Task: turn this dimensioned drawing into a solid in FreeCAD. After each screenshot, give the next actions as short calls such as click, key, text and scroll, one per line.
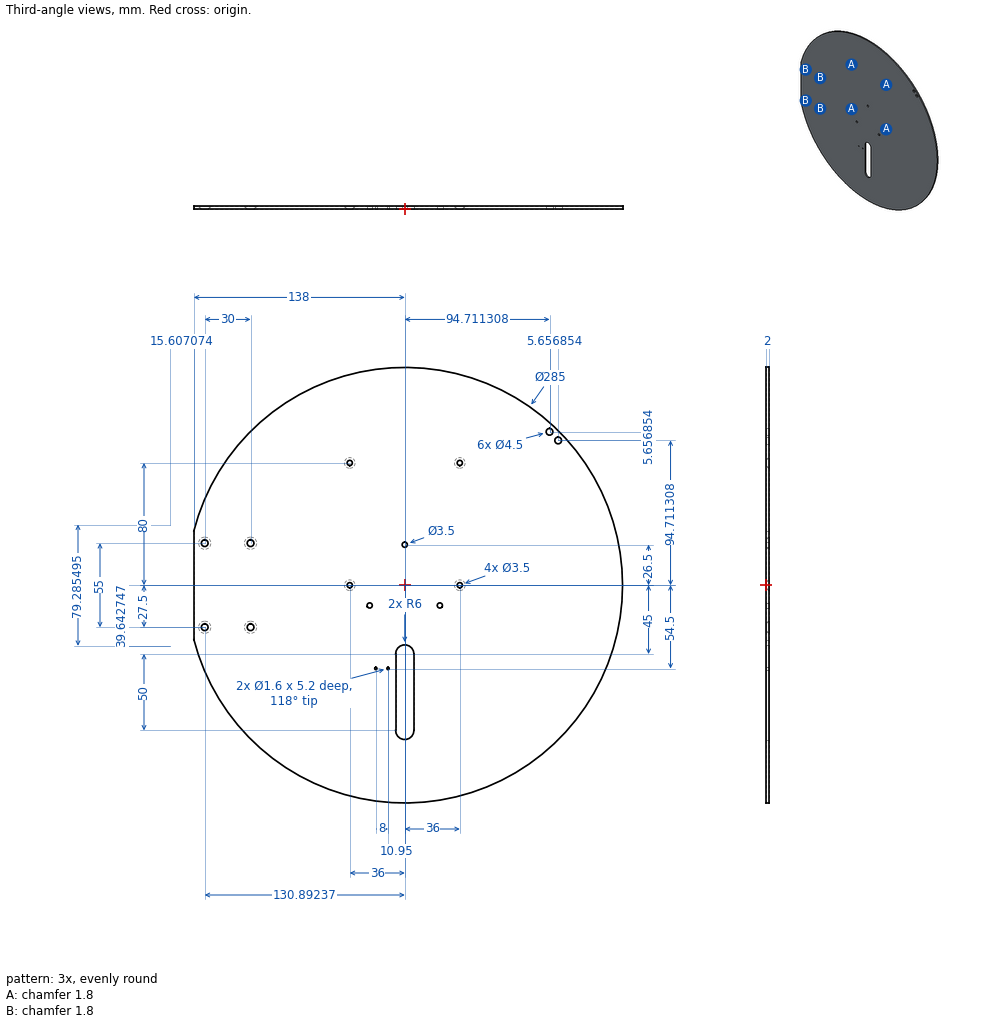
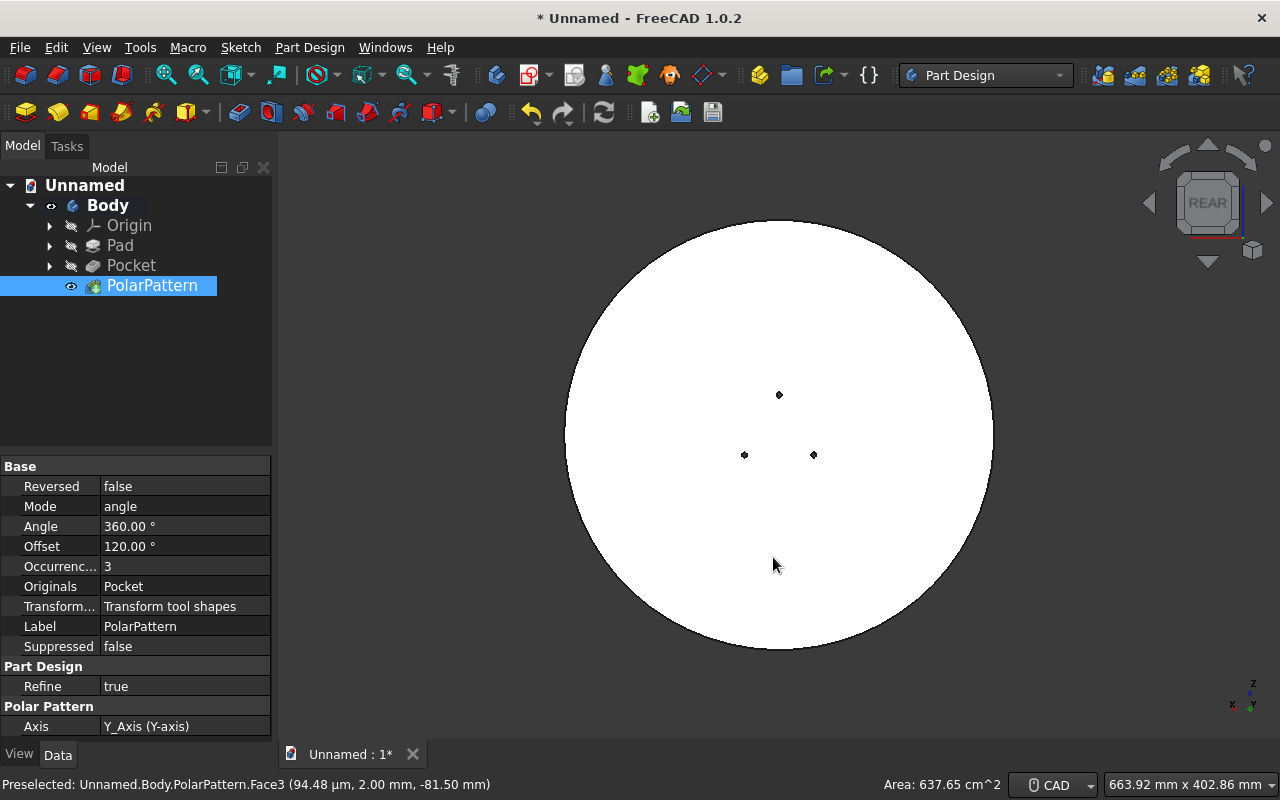
click(530, 76)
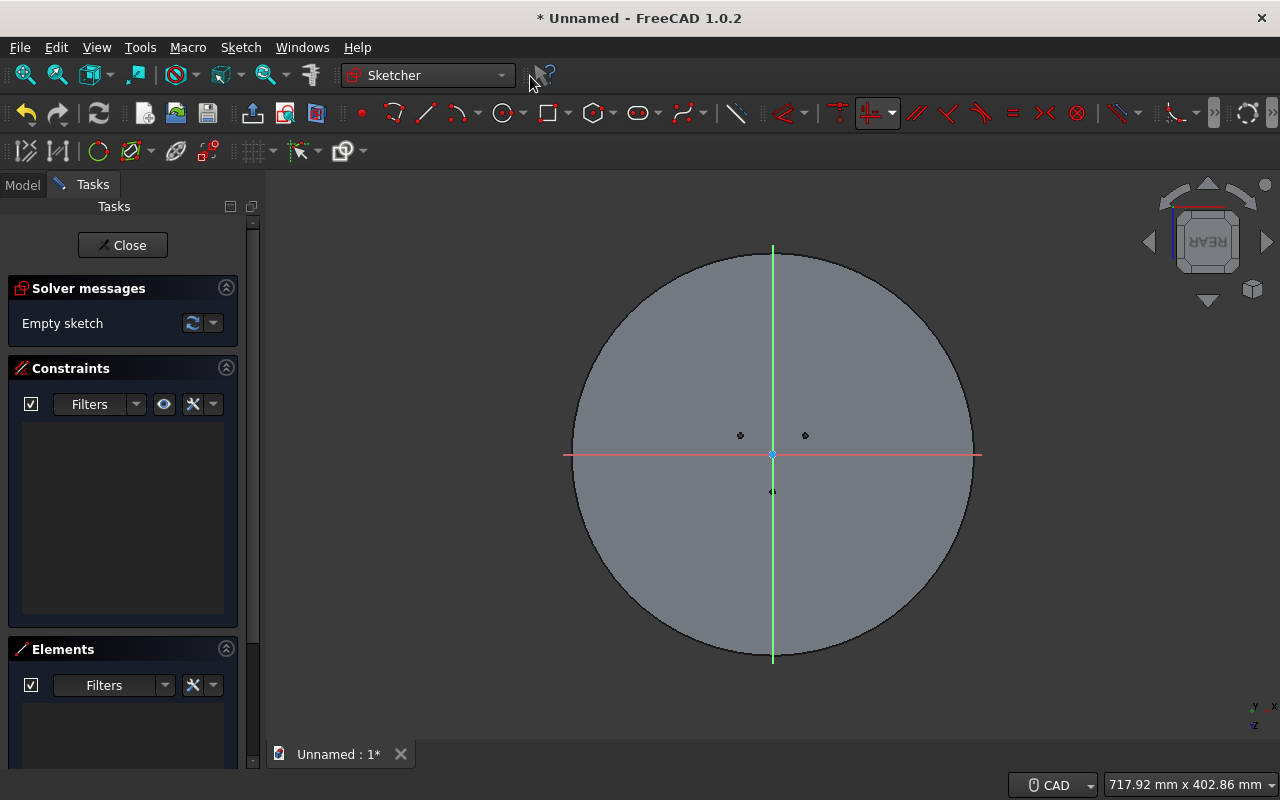
scroll(808, 569, up, 3)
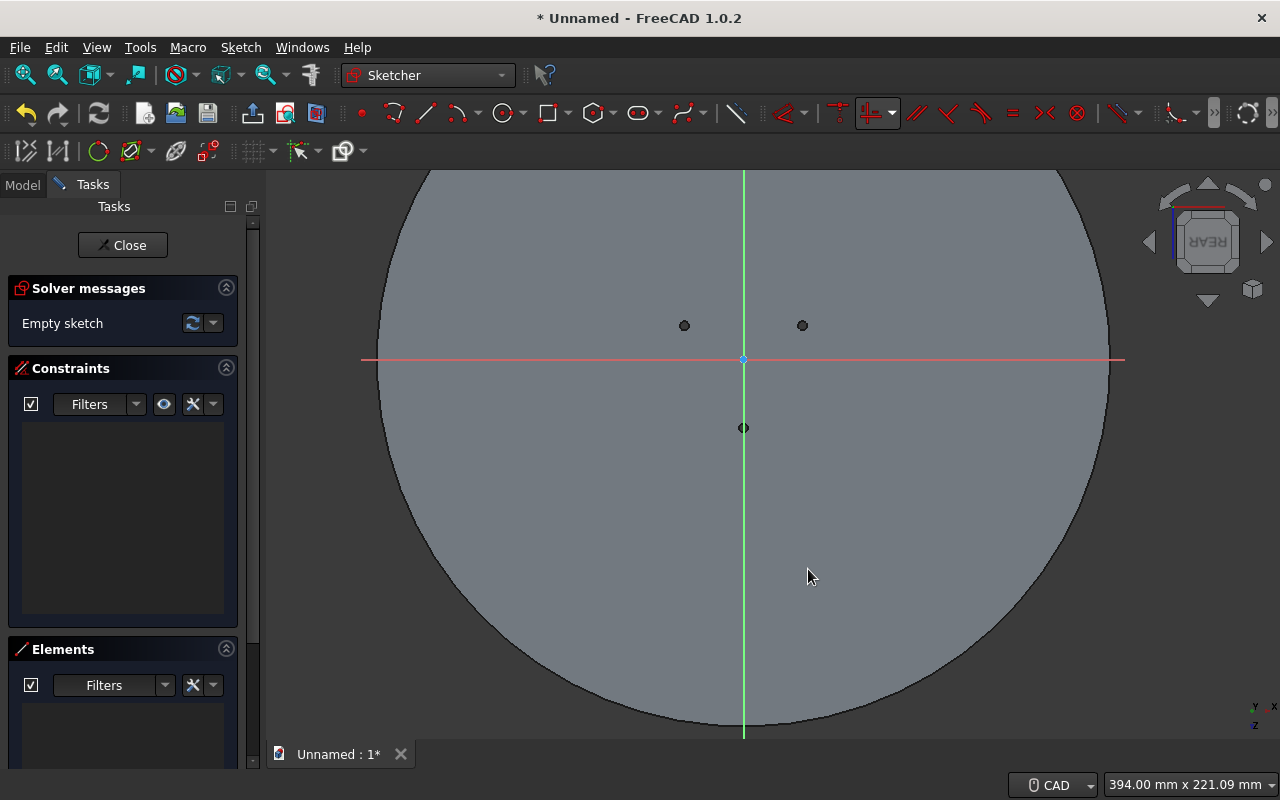
click(504, 114)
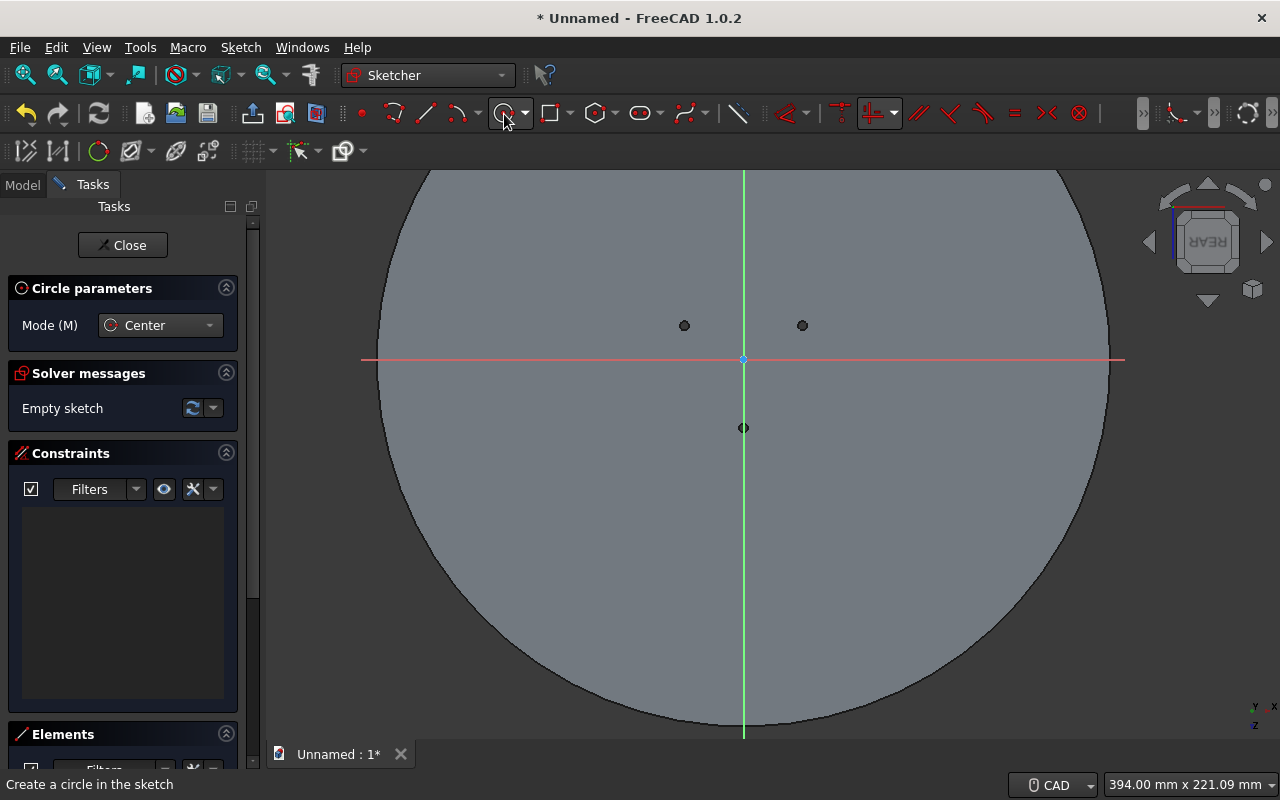
scroll(987, 618, up, 7)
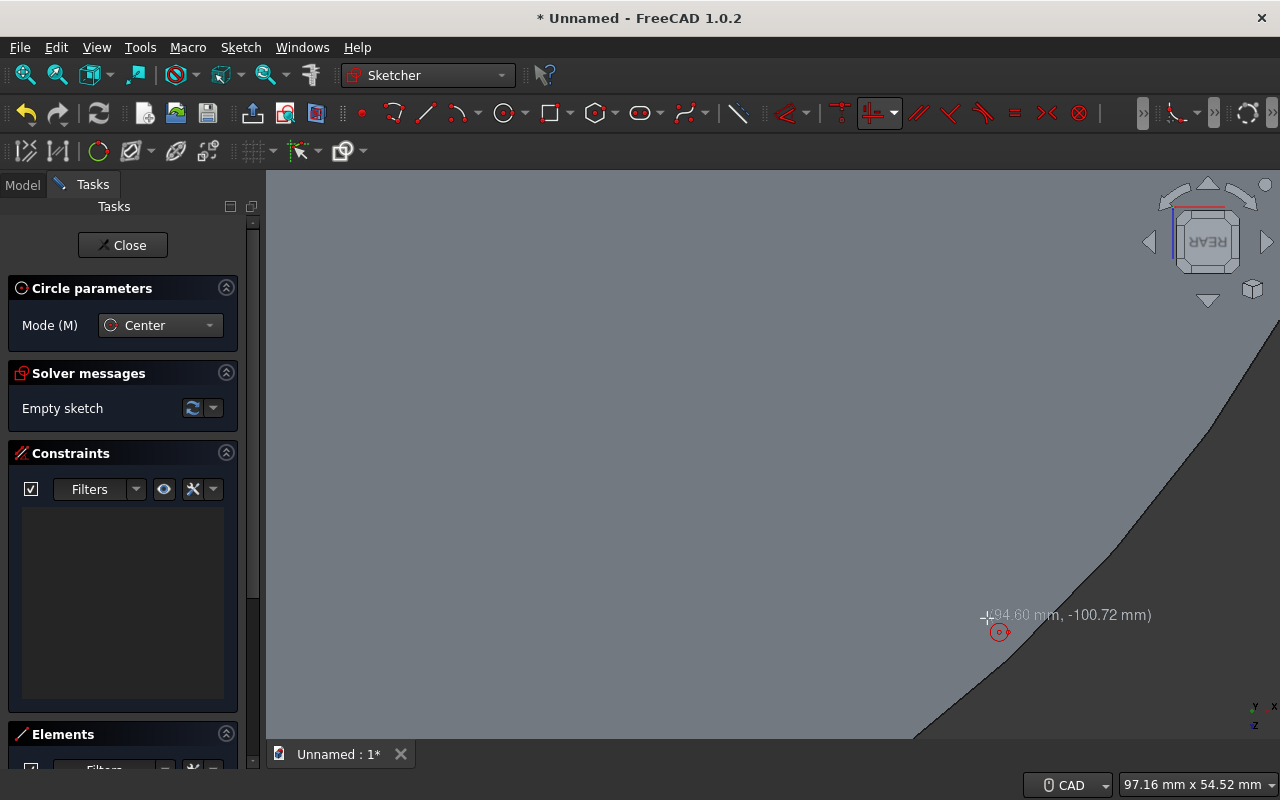
scroll(988, 620, down, 7)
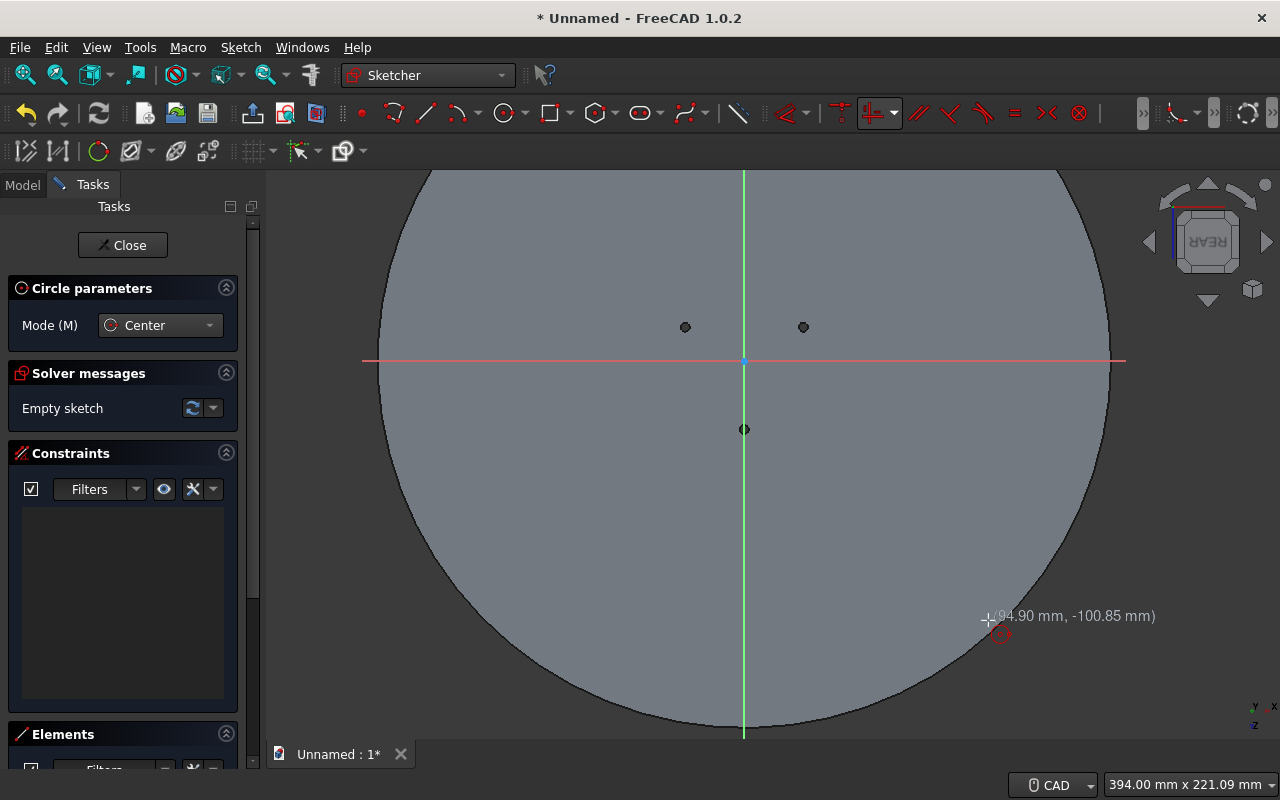
click(988, 620)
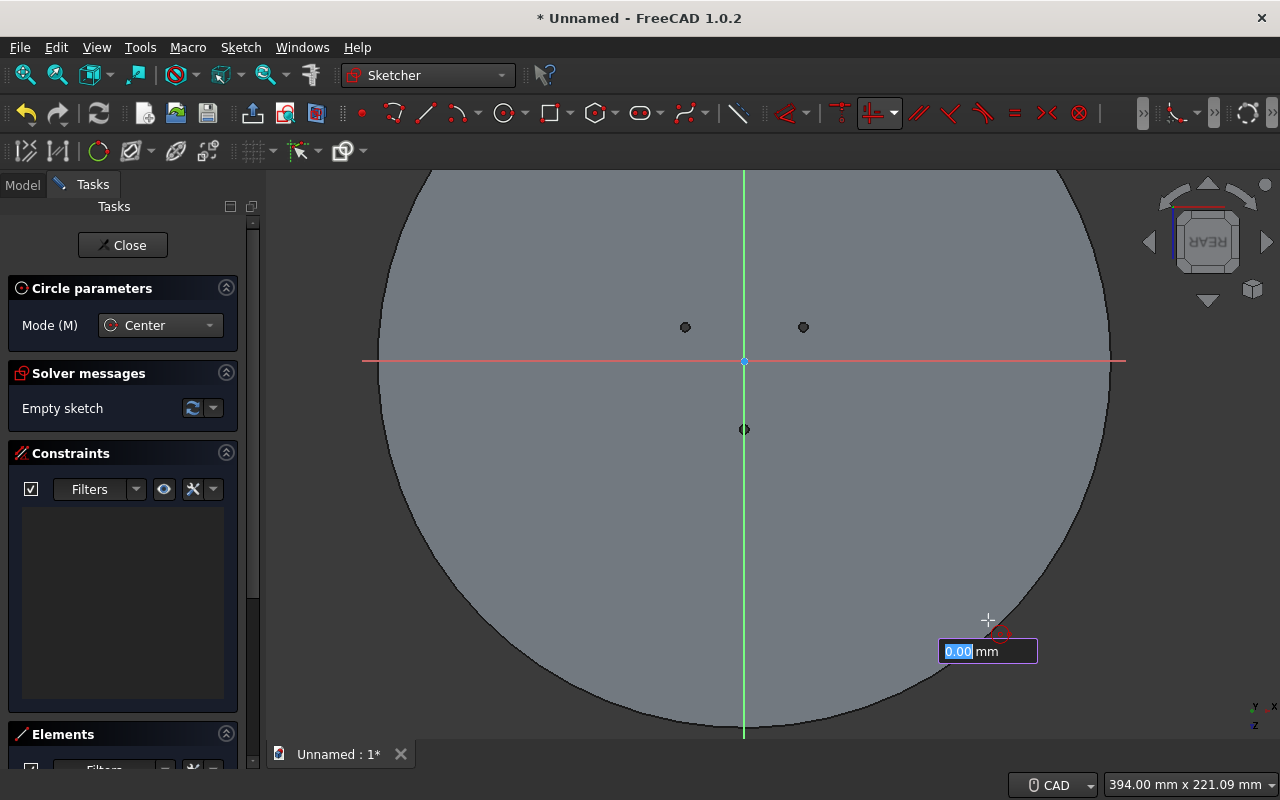
scroll(992, 616, up, 6)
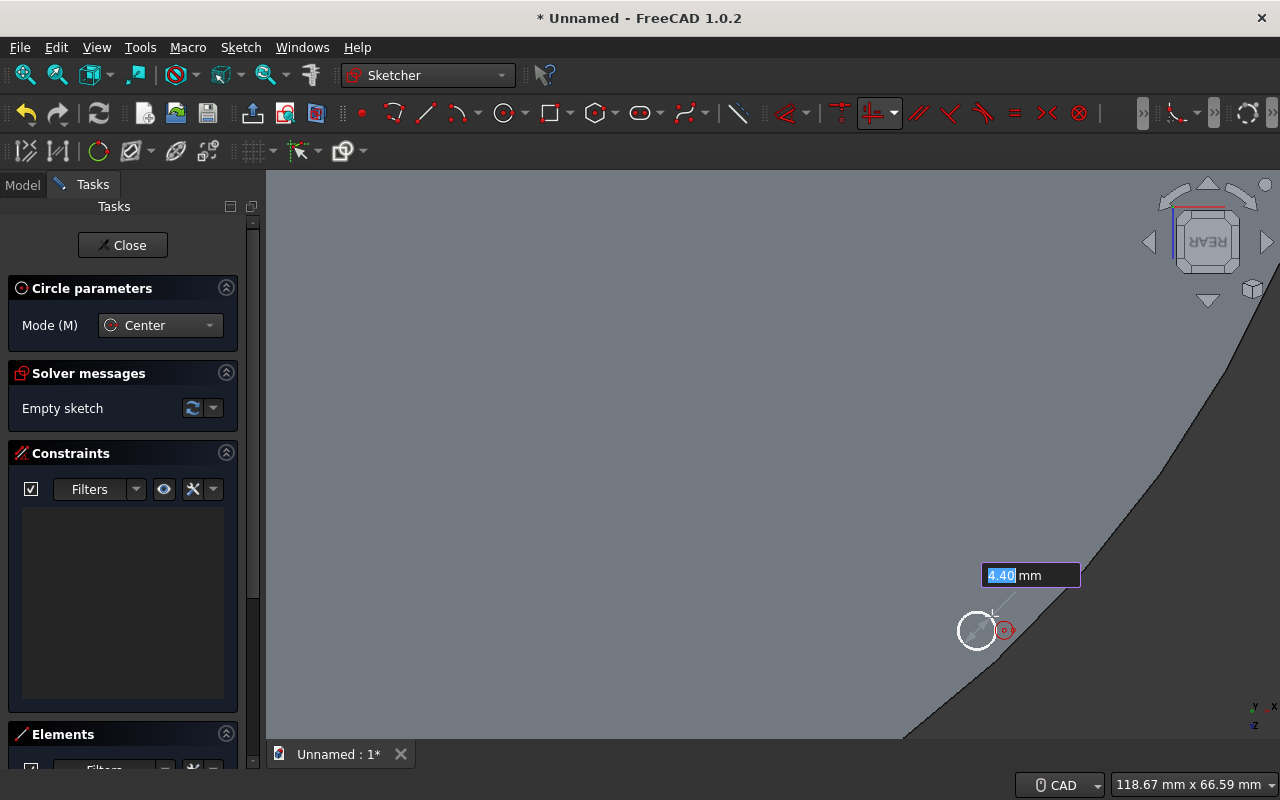
click(991, 613)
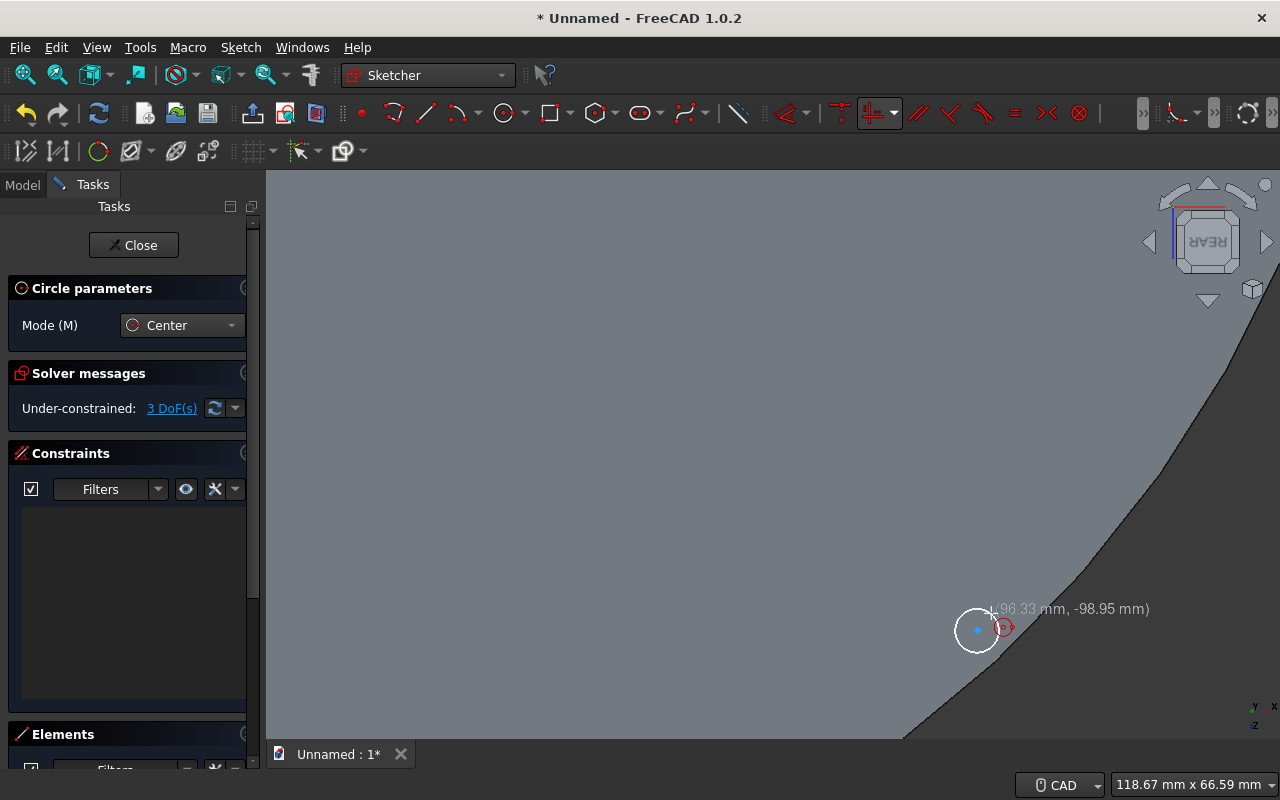
click(1026, 578)
click(1039, 564)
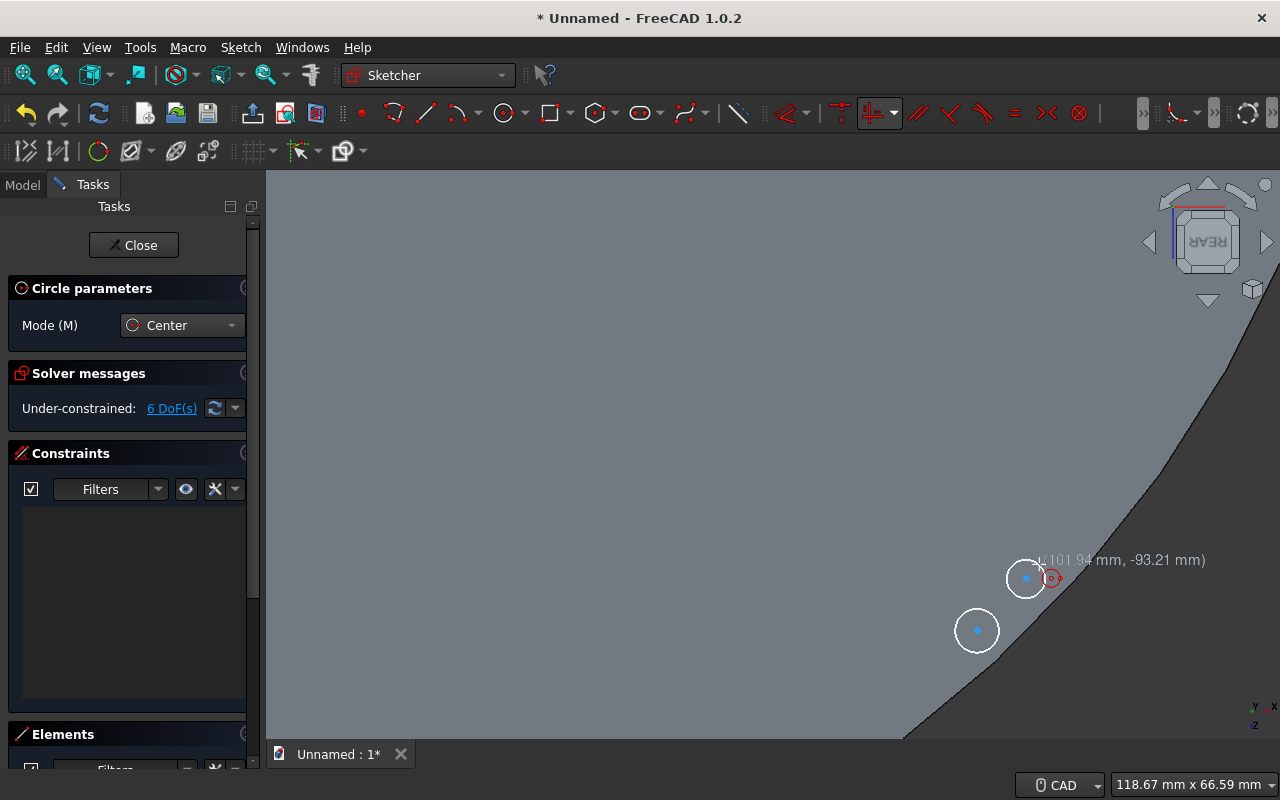
scroll(992, 616, down, 6)